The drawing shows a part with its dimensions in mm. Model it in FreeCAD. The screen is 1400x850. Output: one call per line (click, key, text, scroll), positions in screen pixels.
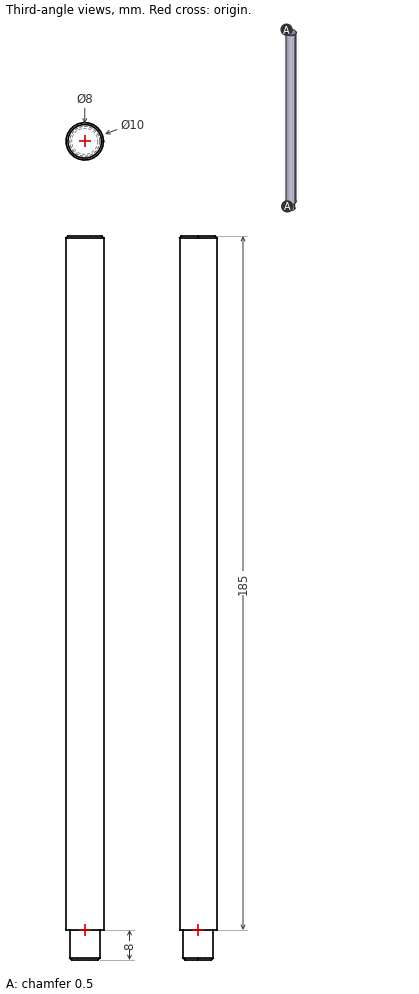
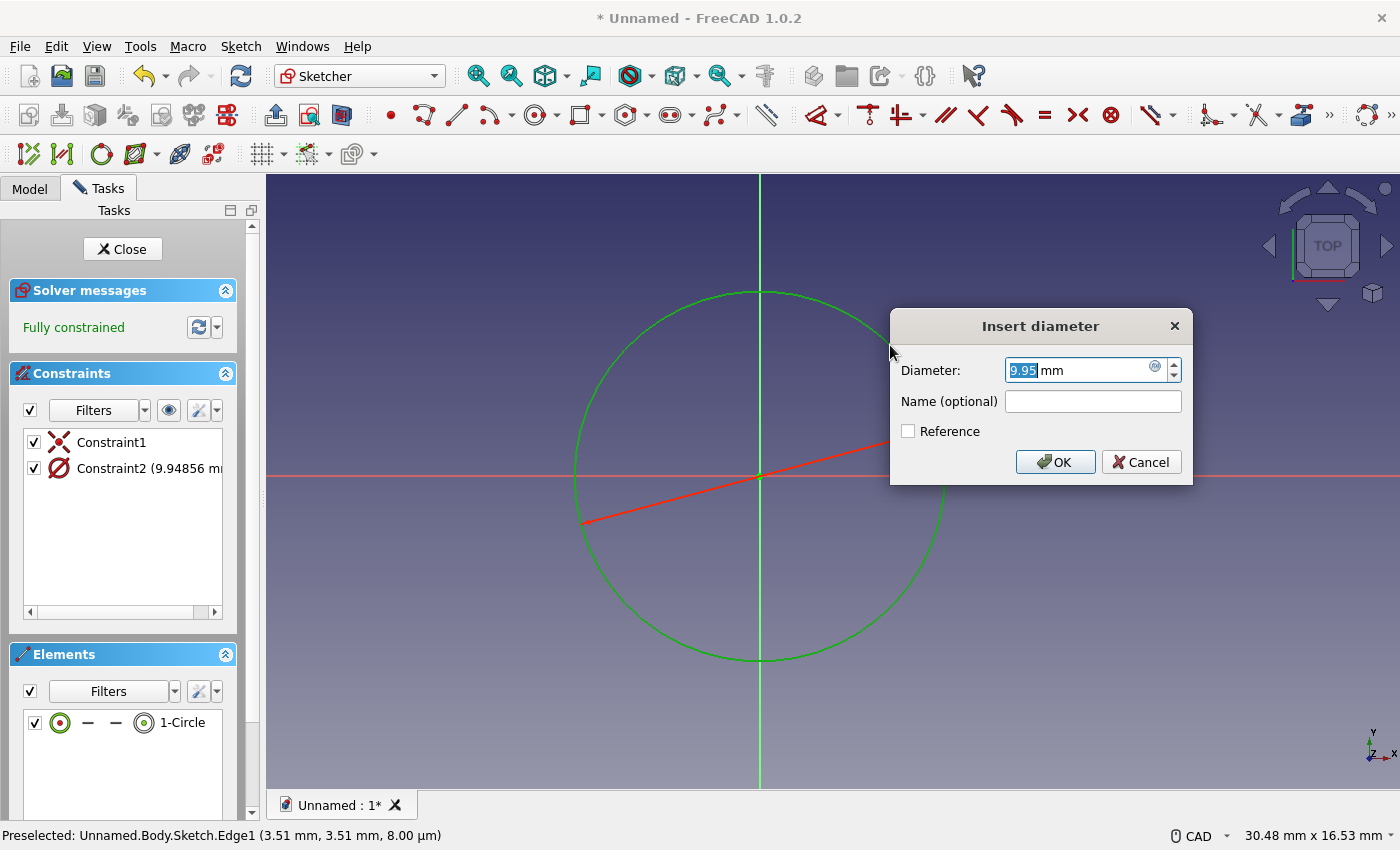
text(10)
key(Return)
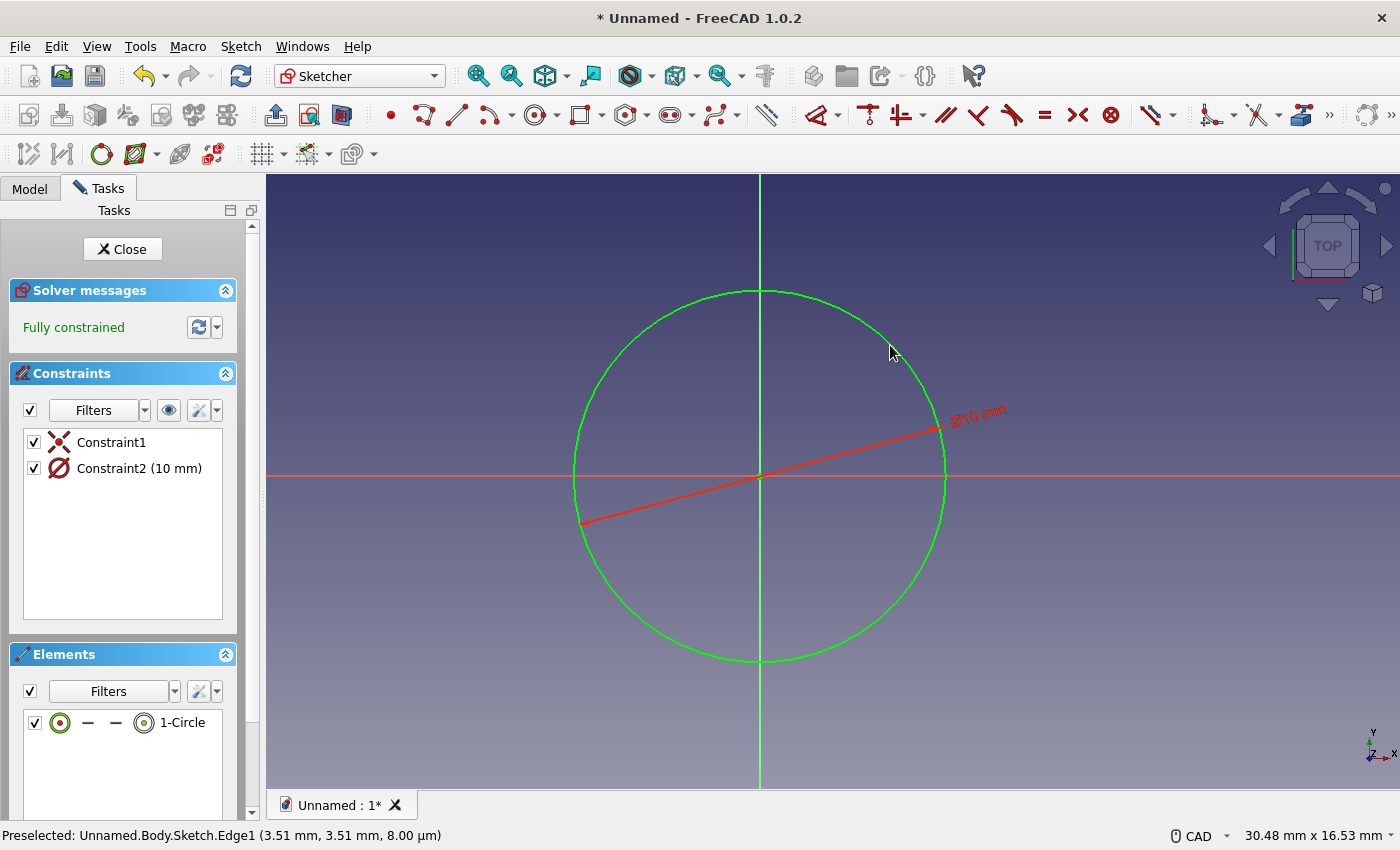
click(123, 249)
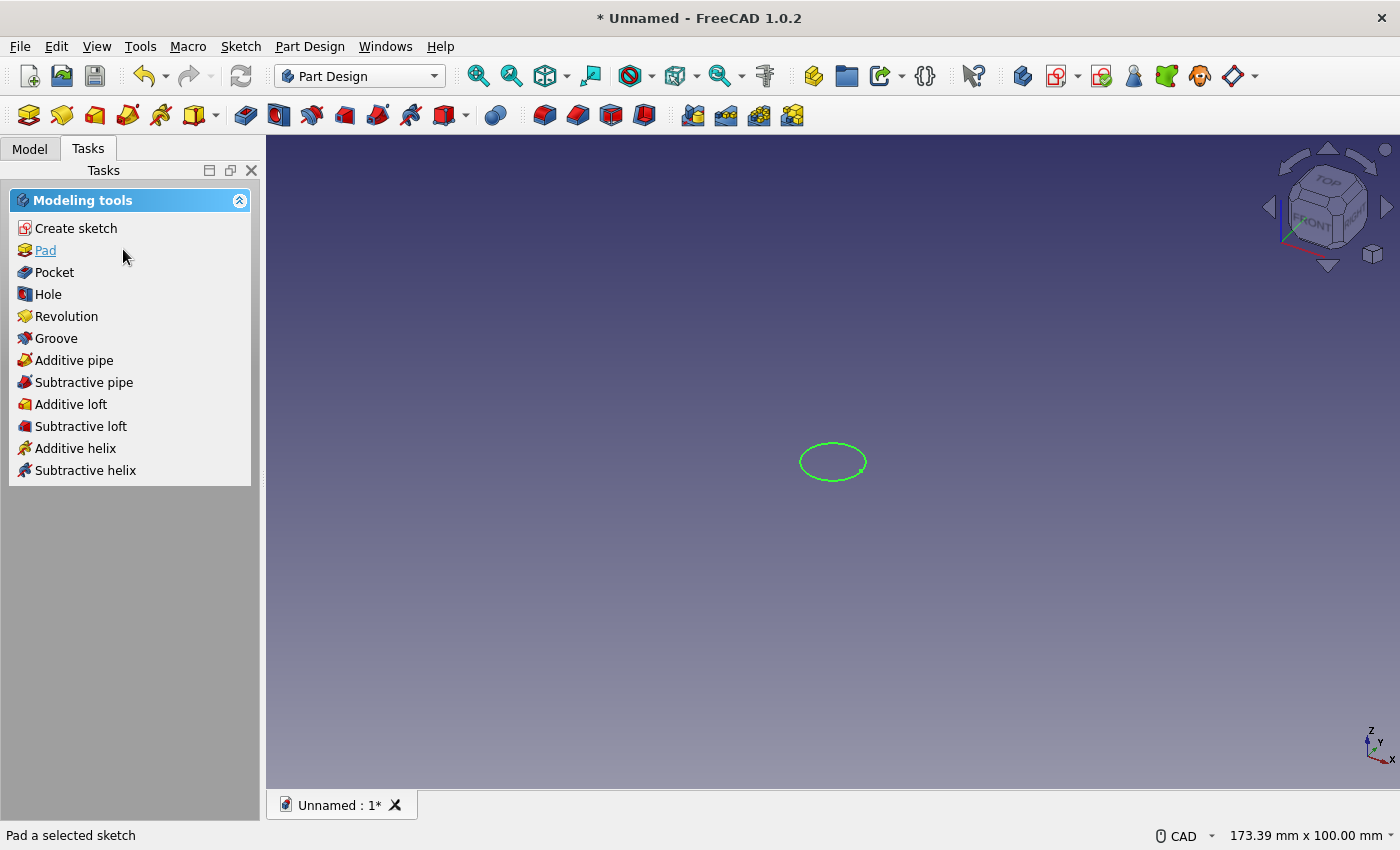
click(29, 116)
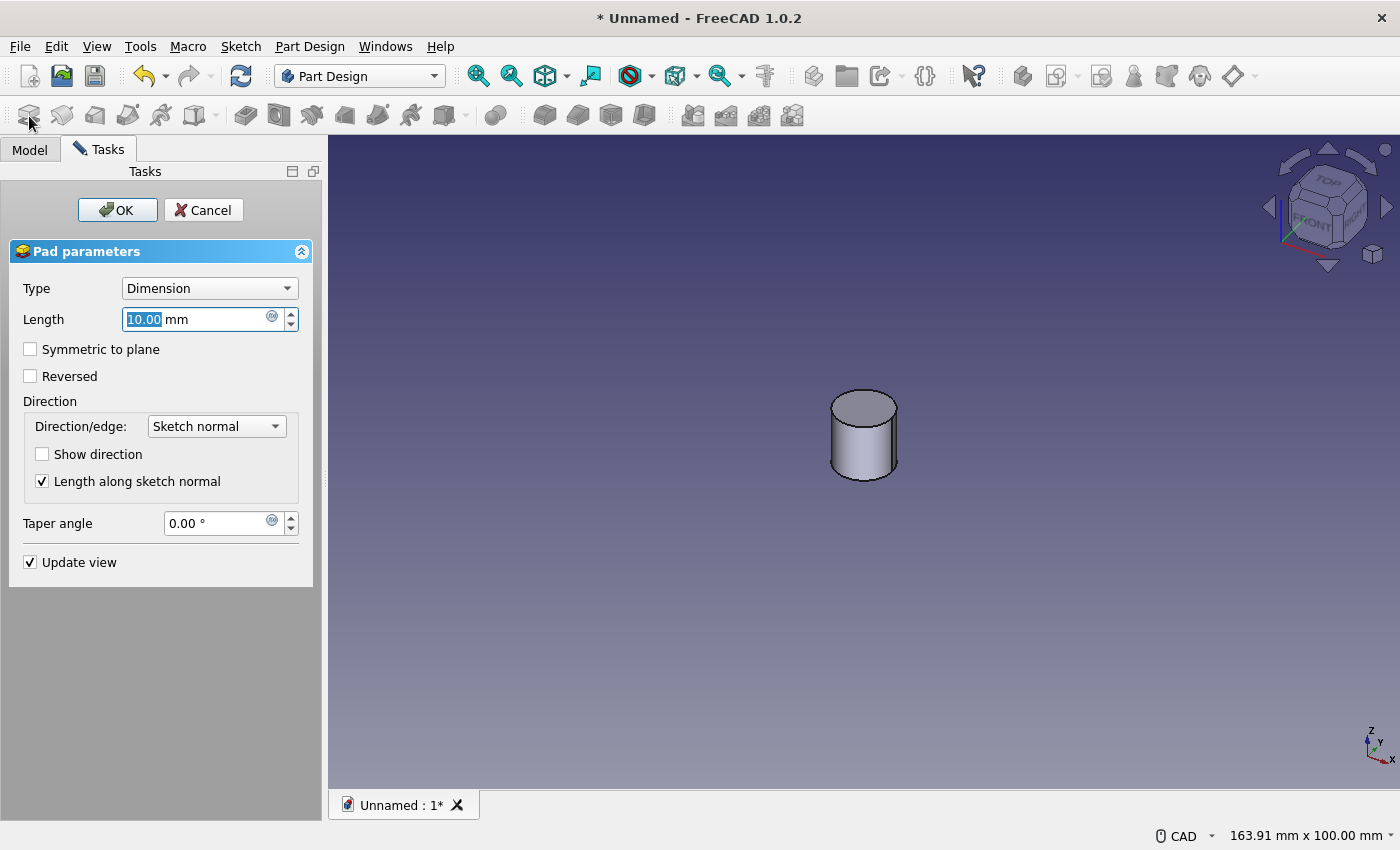
text(185)
key(Tab)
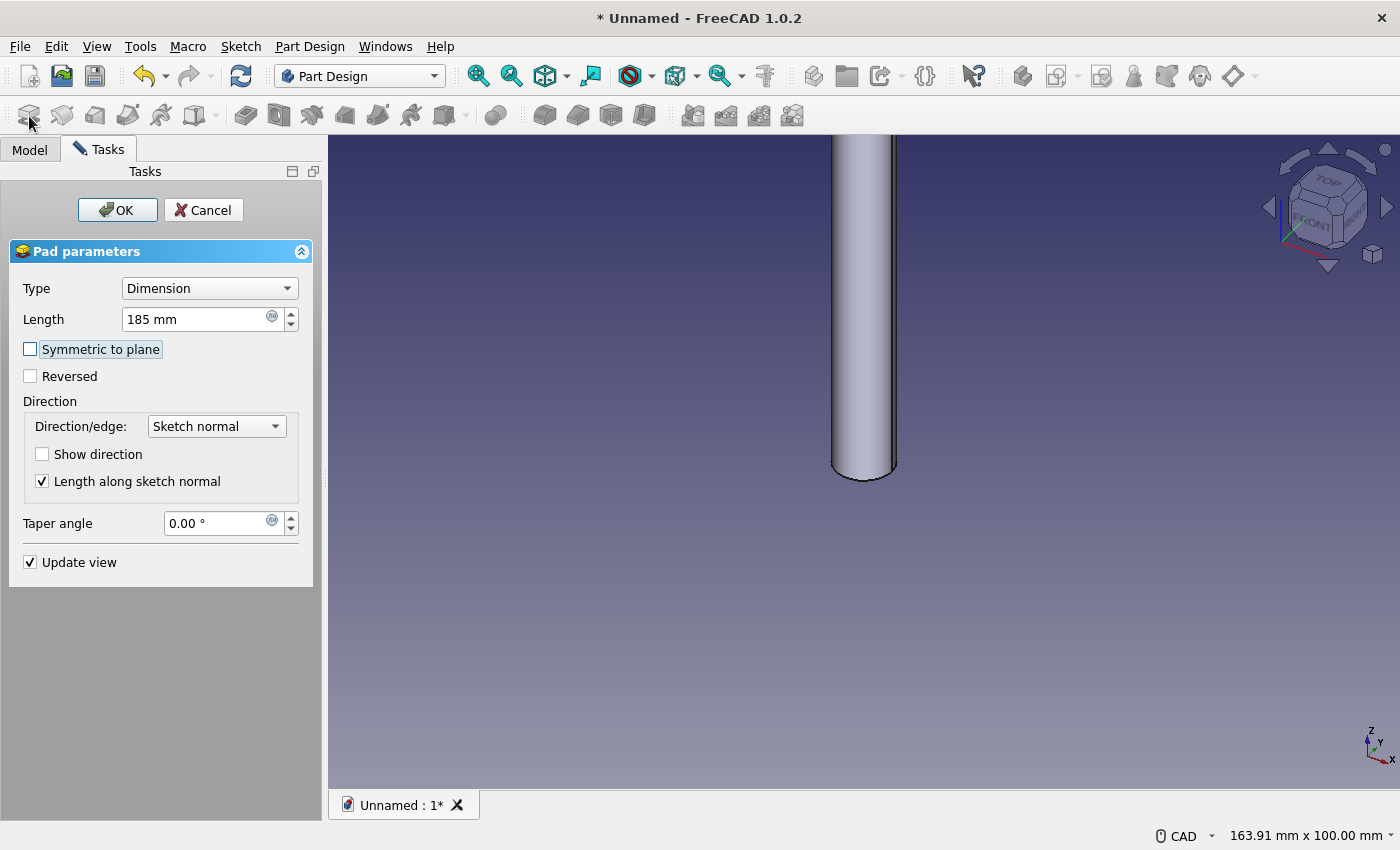
click(118, 210)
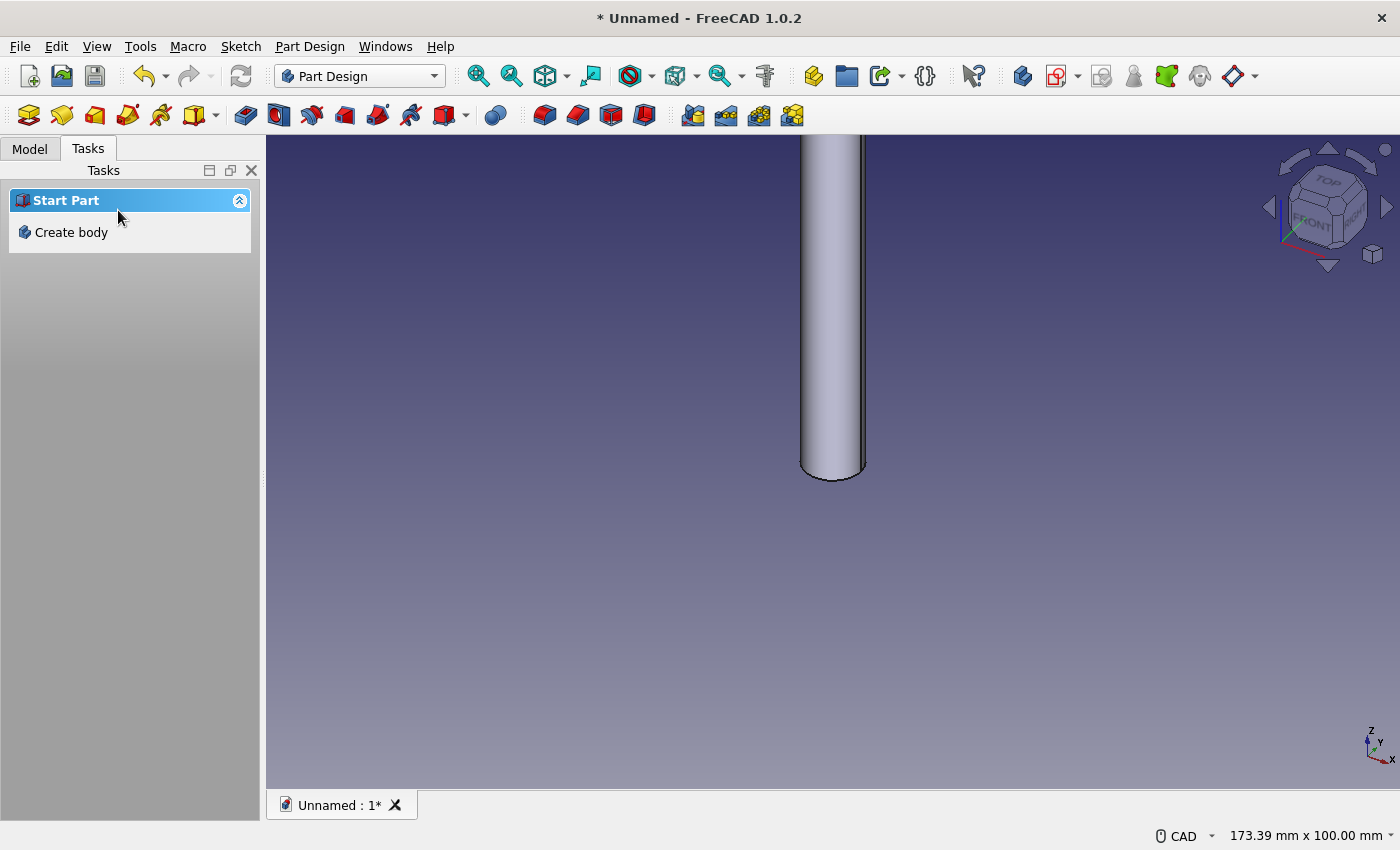
key(v)
key(f)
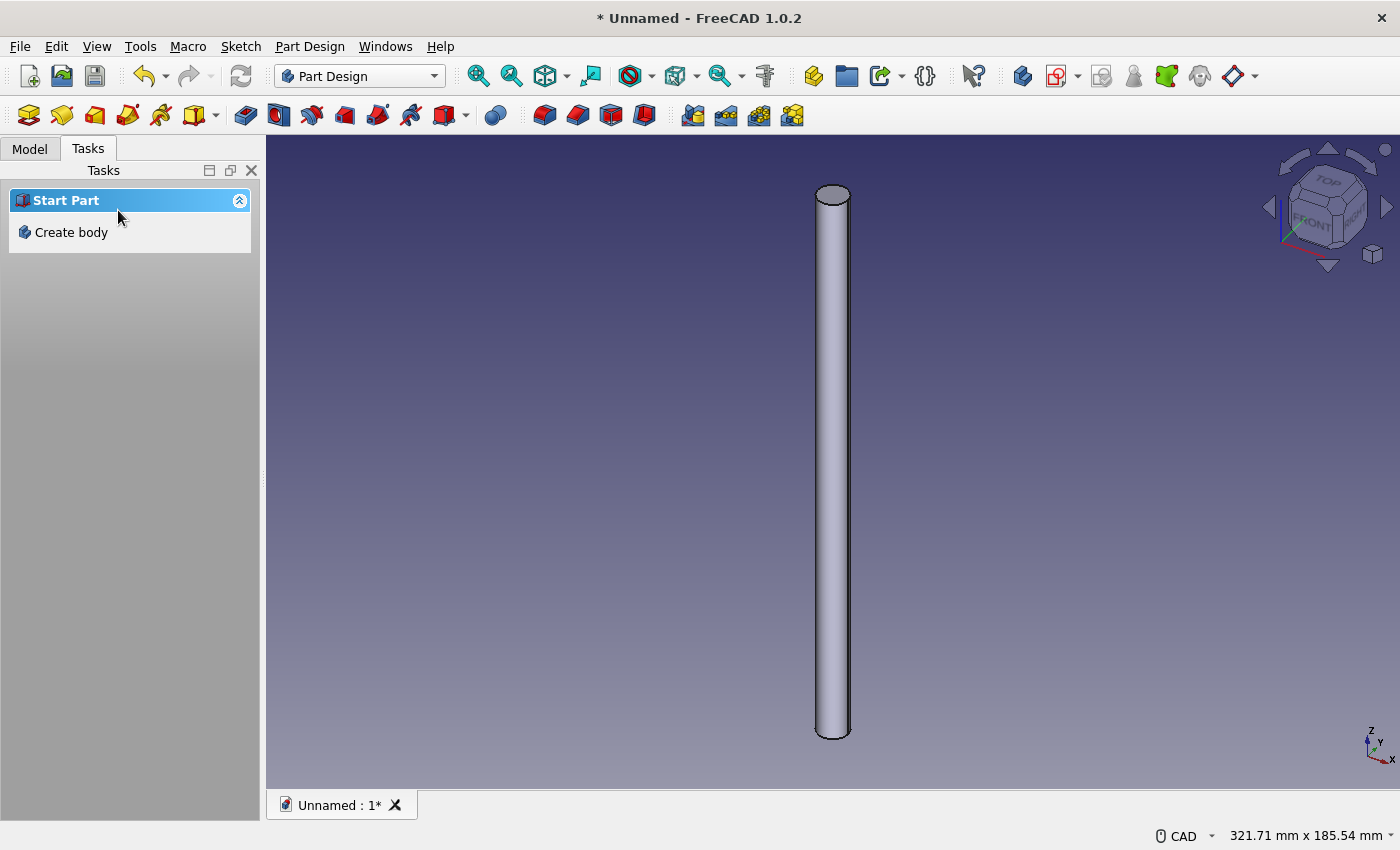
click(1056, 76)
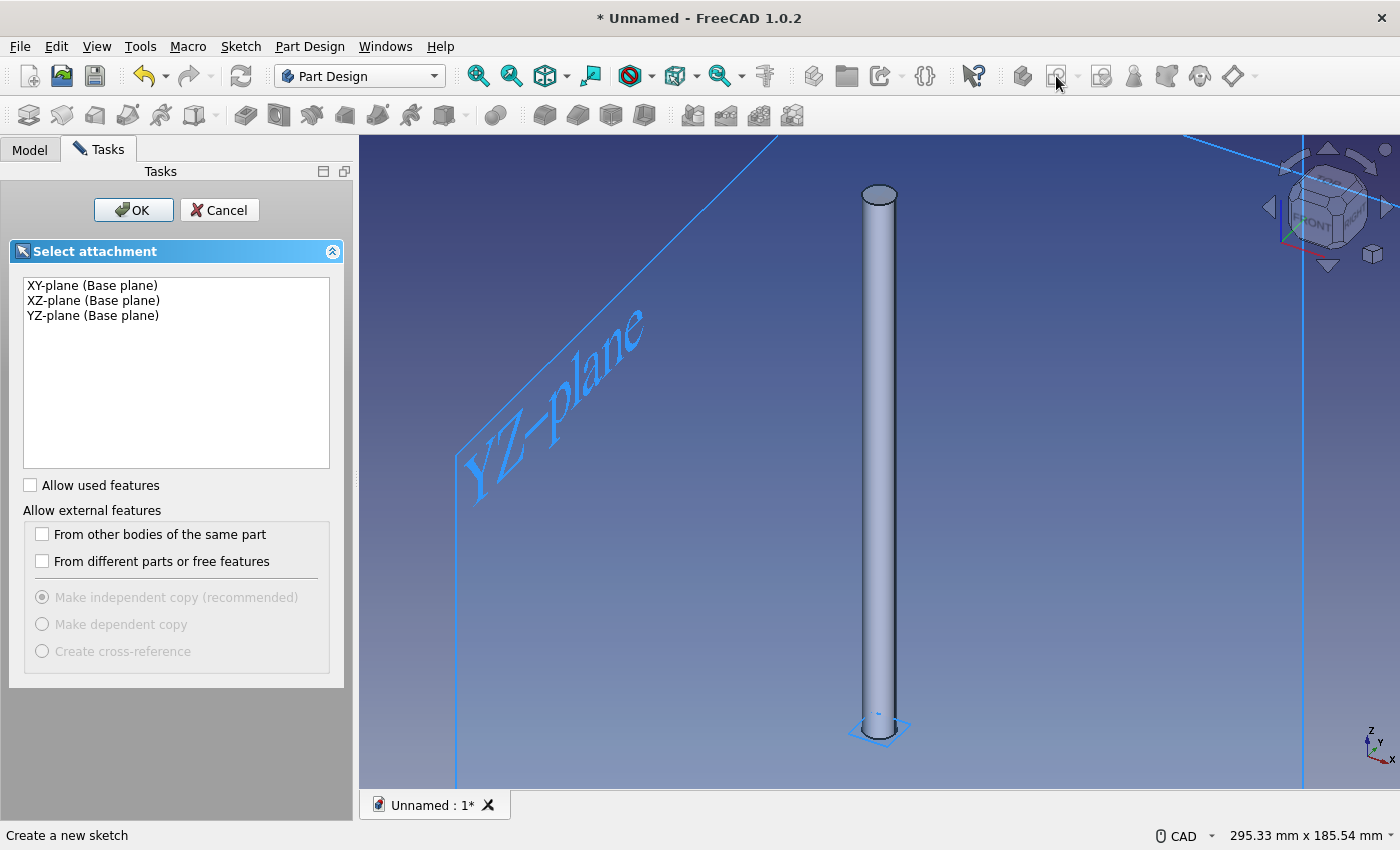
click(84, 286)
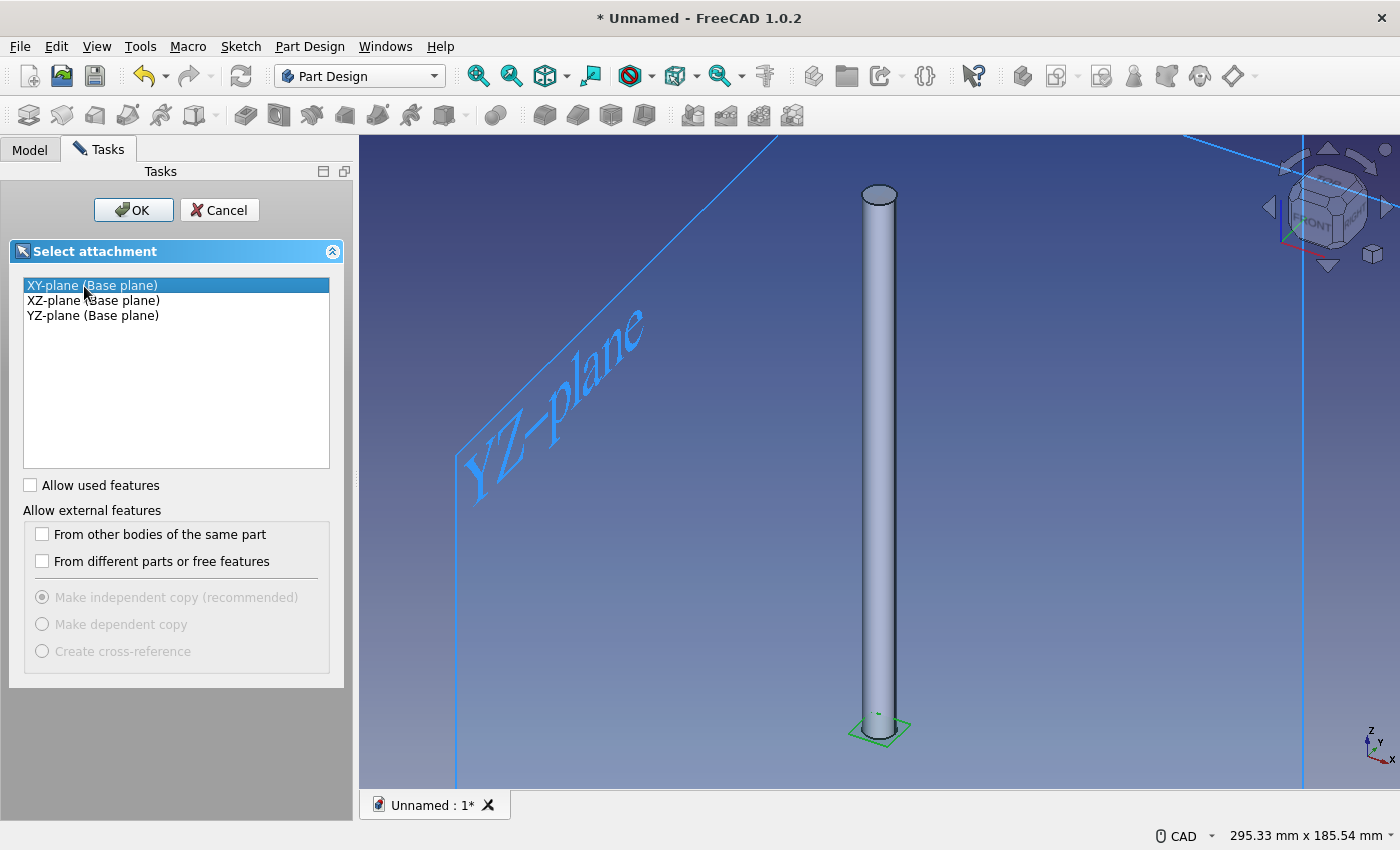
click(134, 210)